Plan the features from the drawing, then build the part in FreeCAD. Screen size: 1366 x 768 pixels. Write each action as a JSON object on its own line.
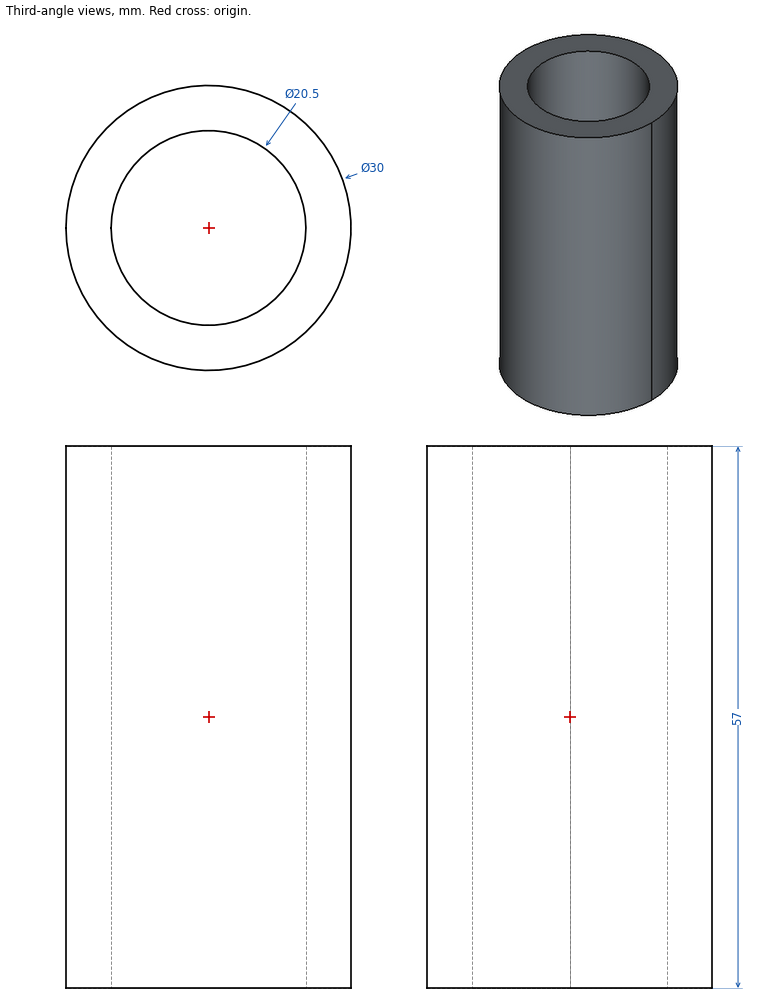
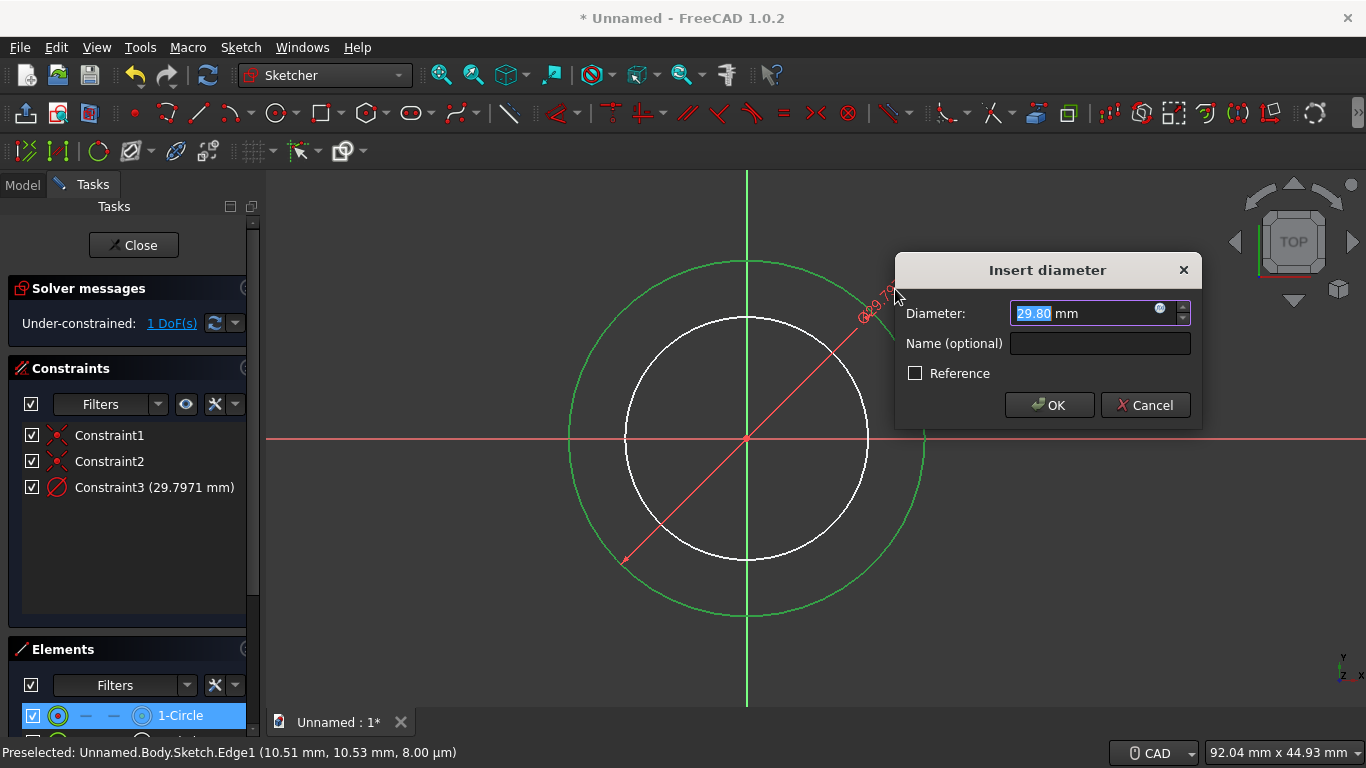
{"action": "type", "text": "30"}
{"action": "key", "text": "Return"}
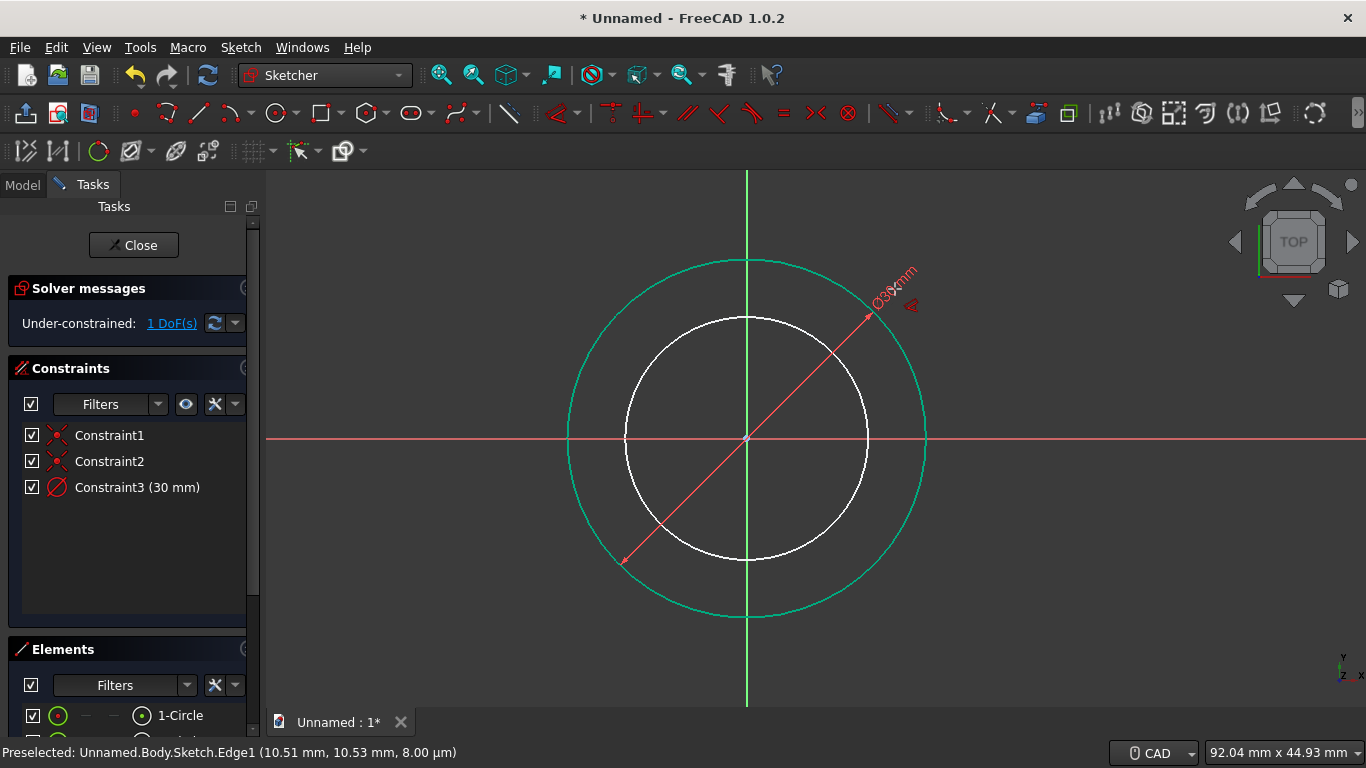
{"action": "left_click", "coordinate": [832, 352]}
{"action": "left_click", "coordinate": [854, 329]}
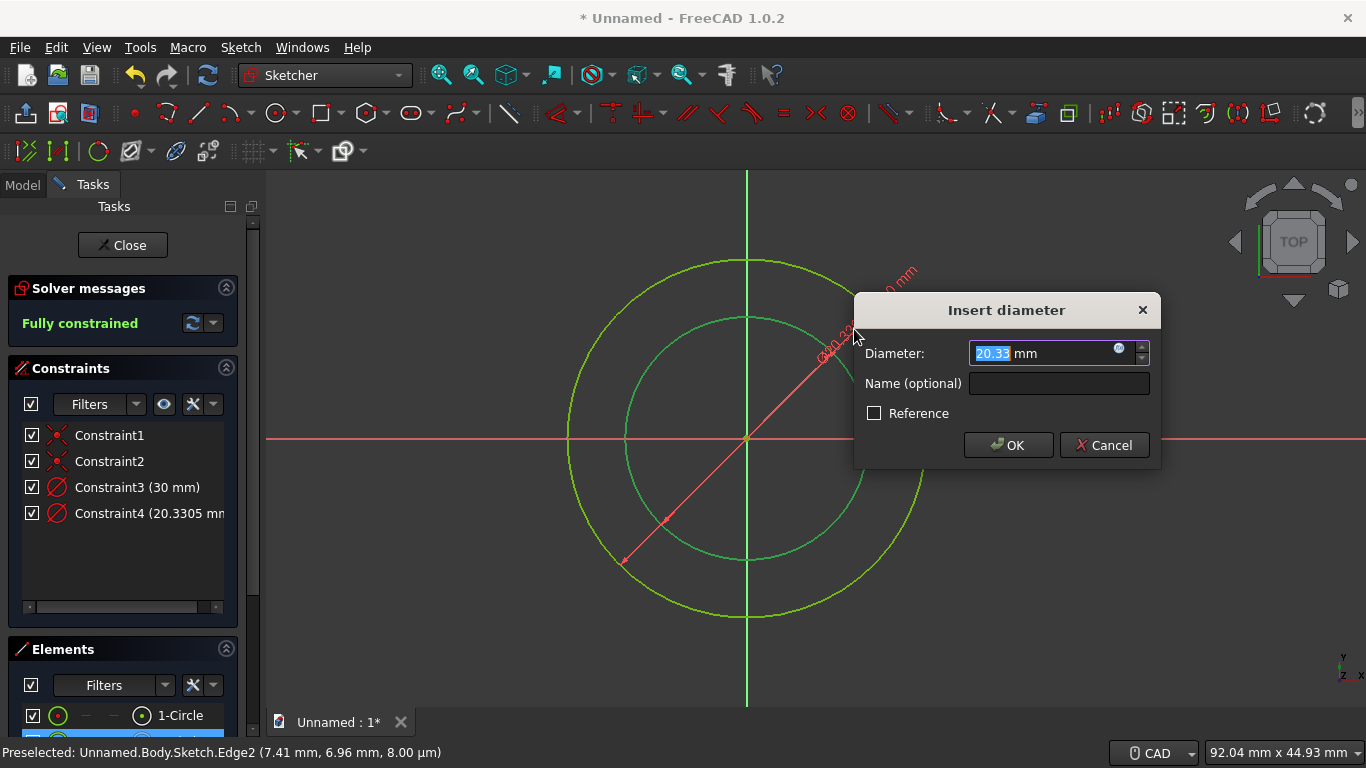
{"action": "type", "text": "20.5"}
{"action": "key", "text": "Return"}
{"action": "key", "text": "Escape"}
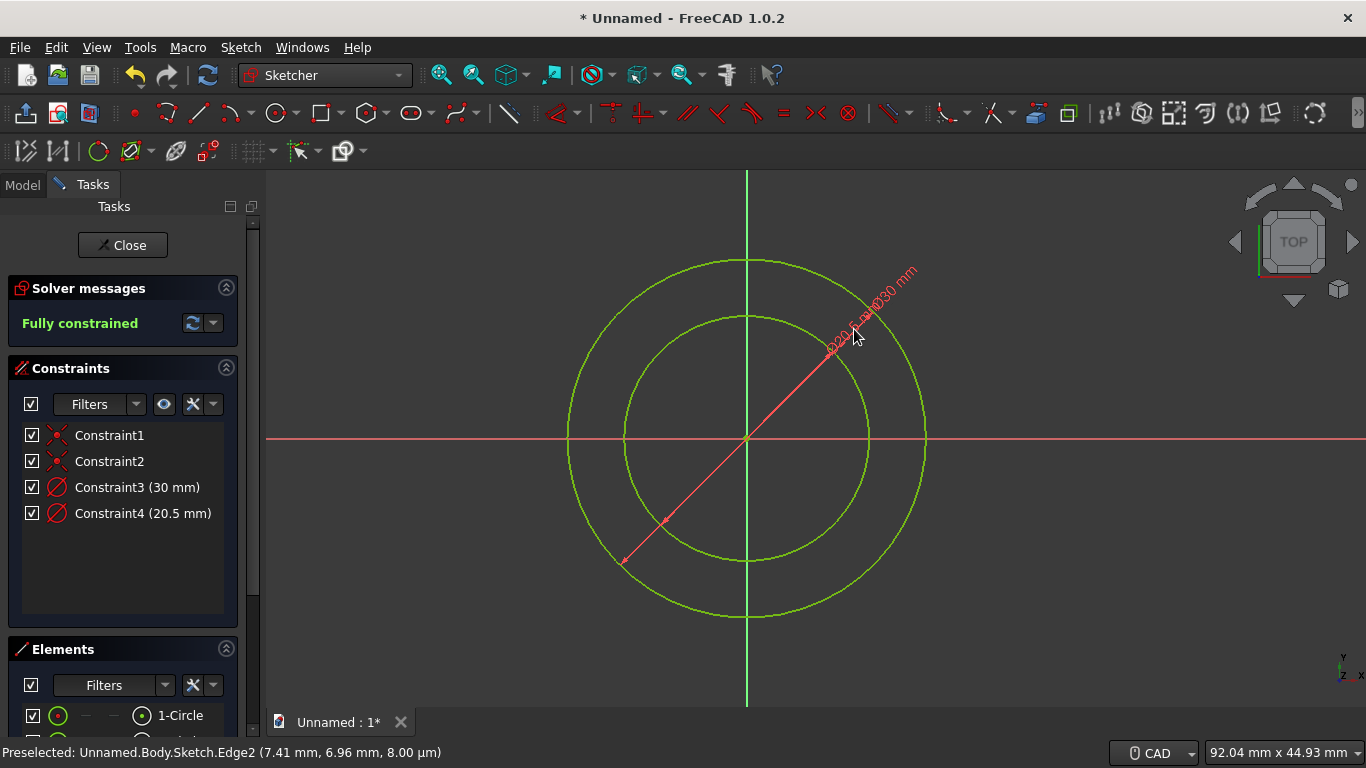
{"action": "left_click", "coordinate": [123, 245]}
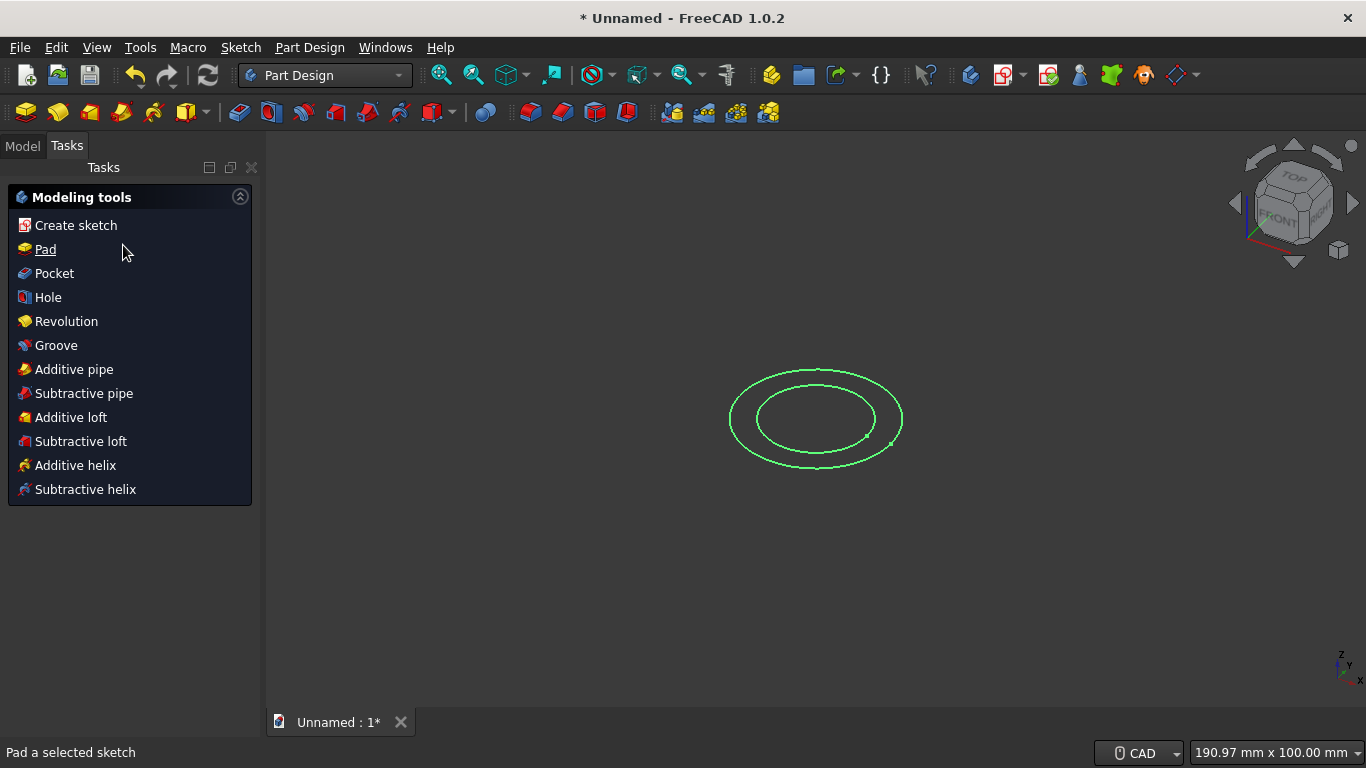
{"action": "left_click", "coordinate": [26, 112]}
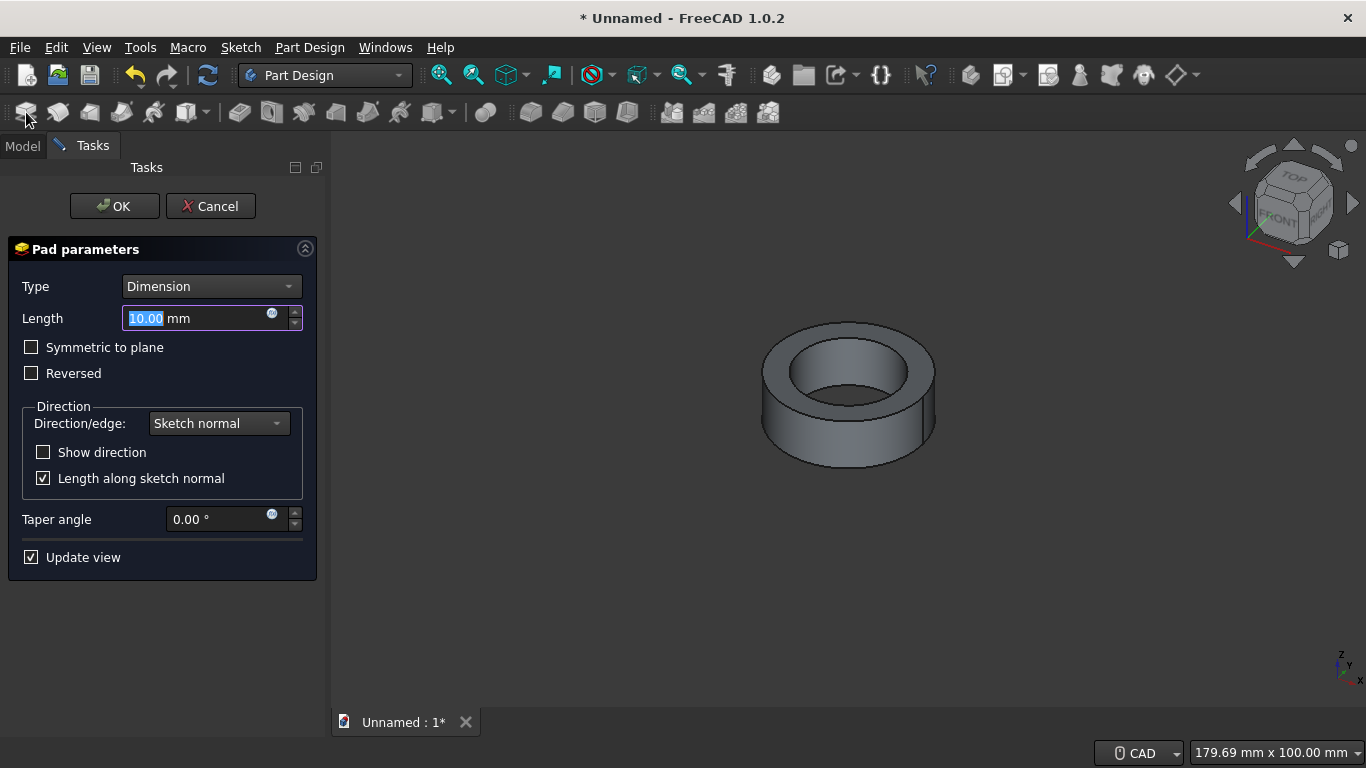
{"action": "type", "text": "57"}
{"action": "key", "text": "Tab"}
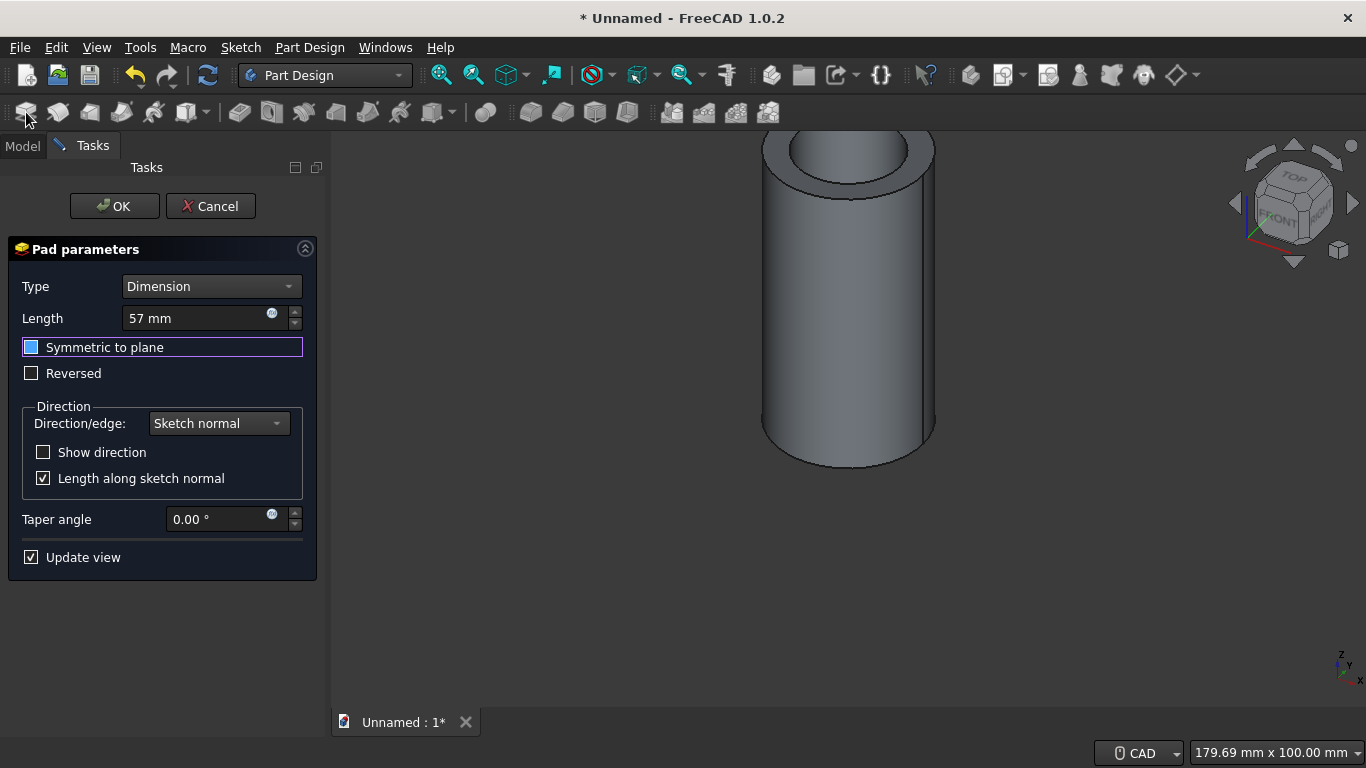
{"action": "left_click", "coordinate": [30, 347]}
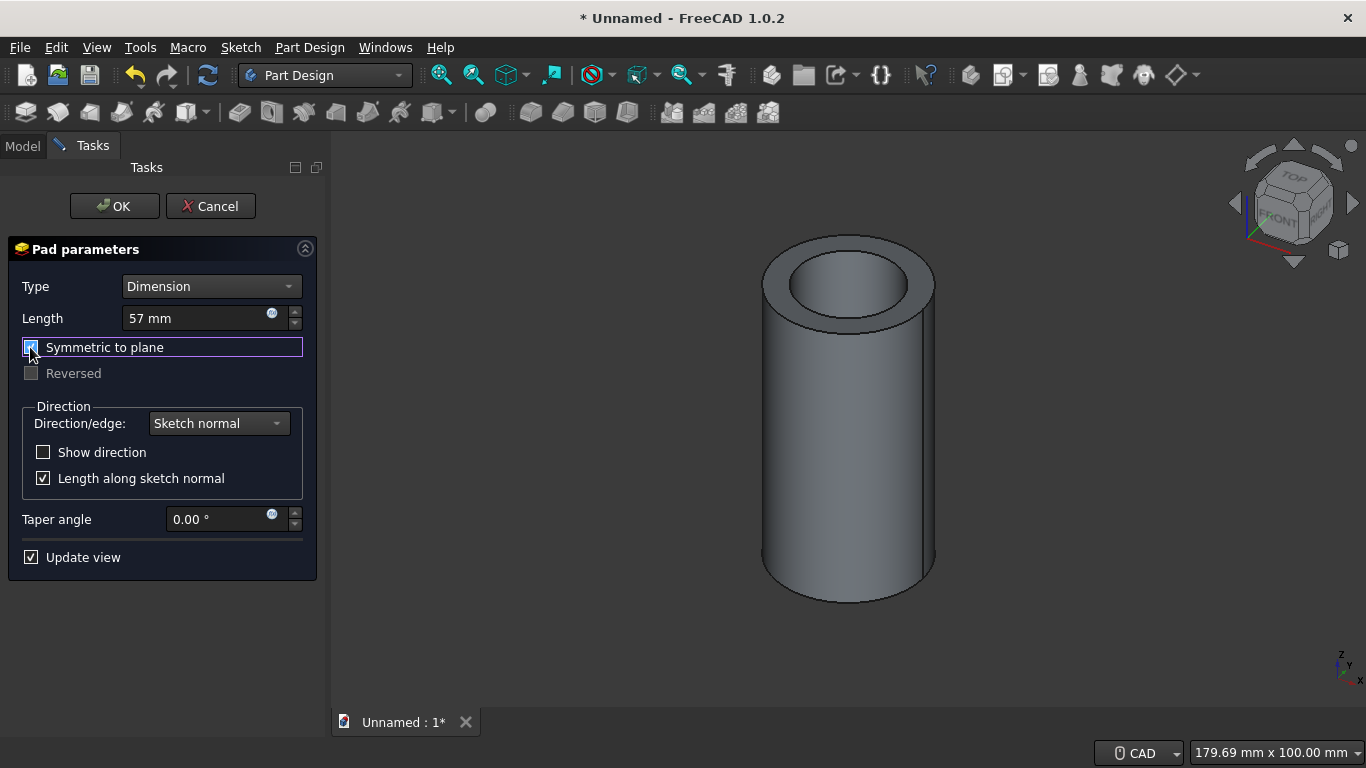
{"action": "left_click", "coordinate": [115, 206]}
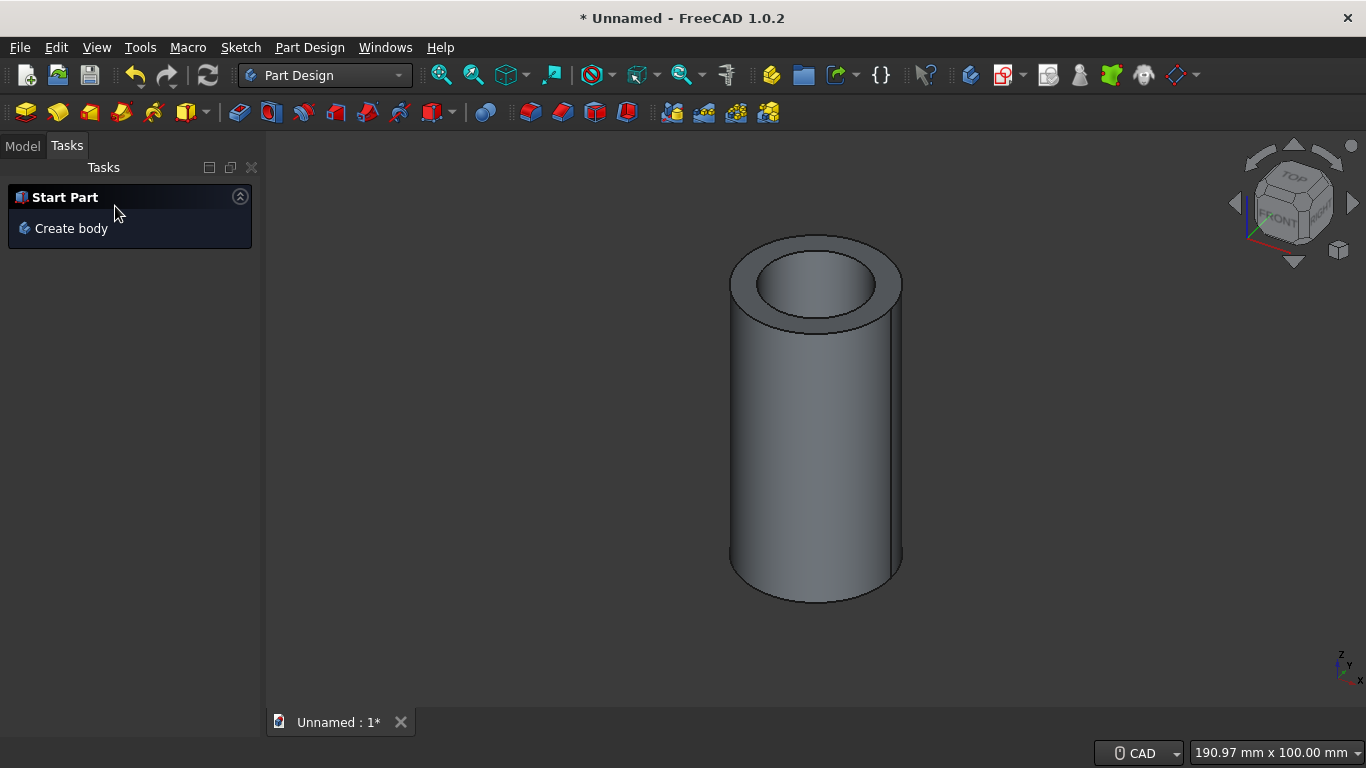
{"action": "key", "text": "0"}